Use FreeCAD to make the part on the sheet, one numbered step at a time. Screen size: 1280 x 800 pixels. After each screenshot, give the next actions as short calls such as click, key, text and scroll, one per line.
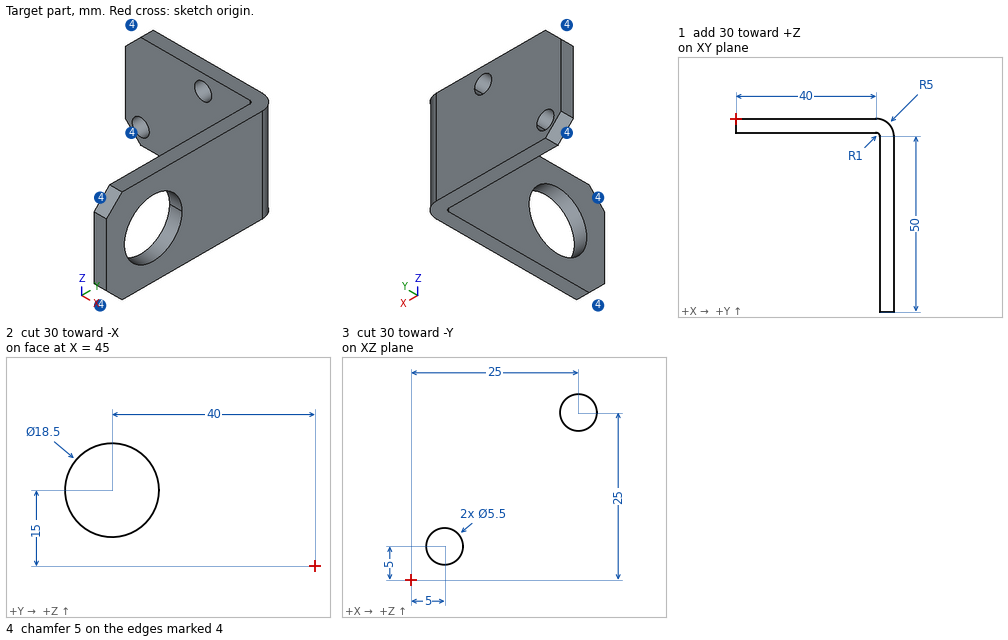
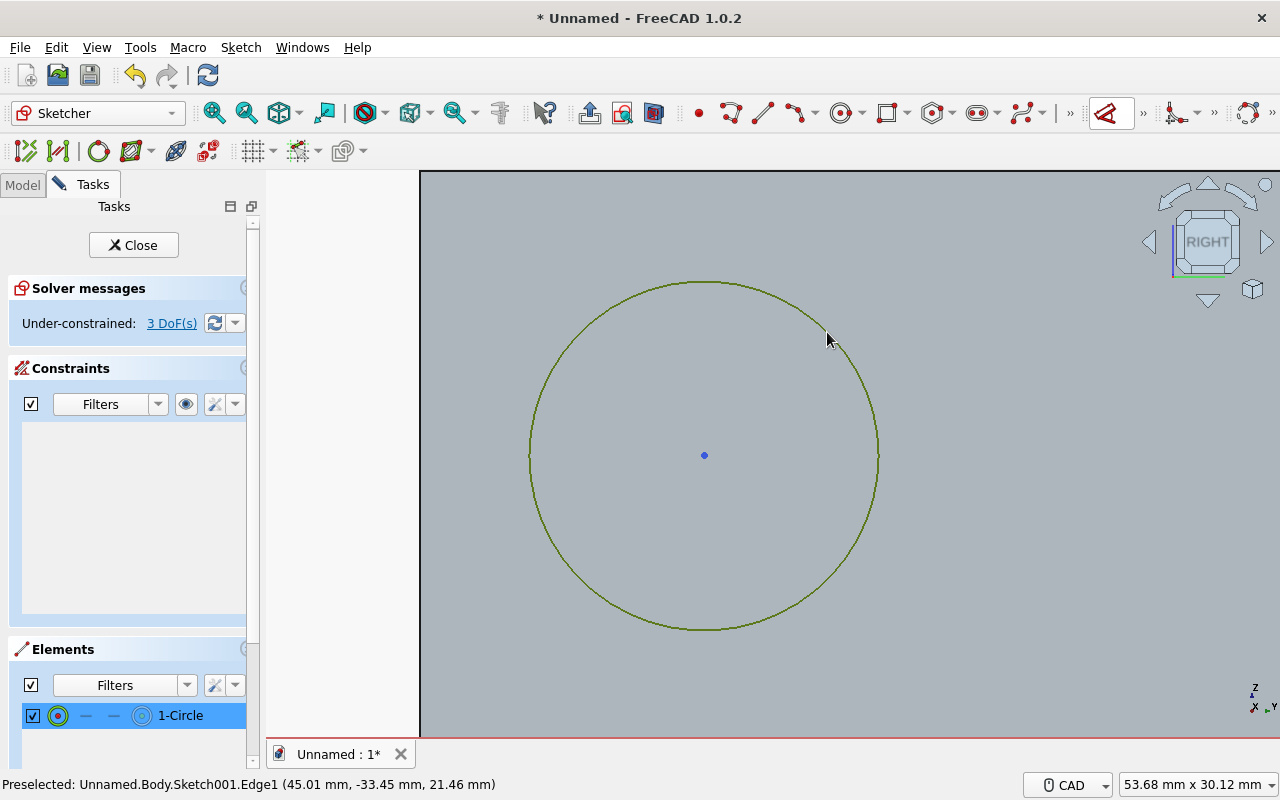
click(1128, 114)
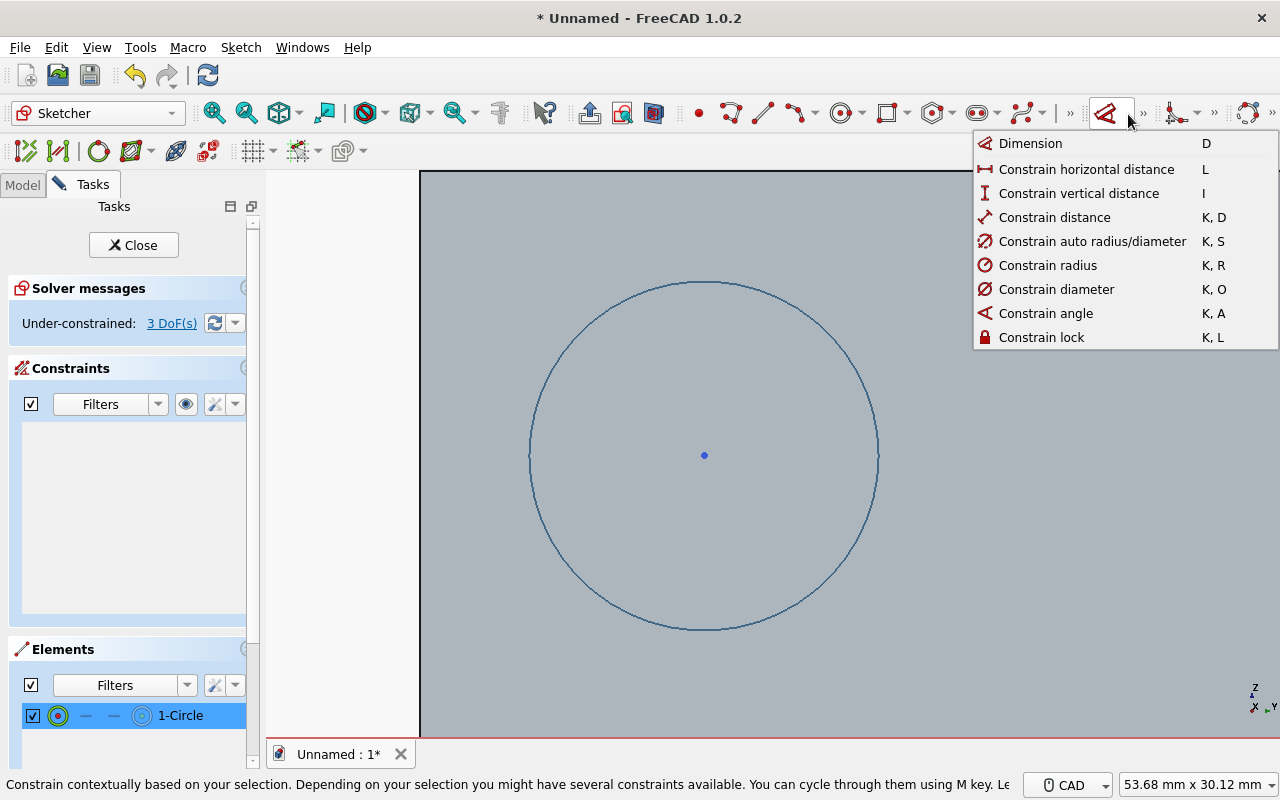
click(1126, 289)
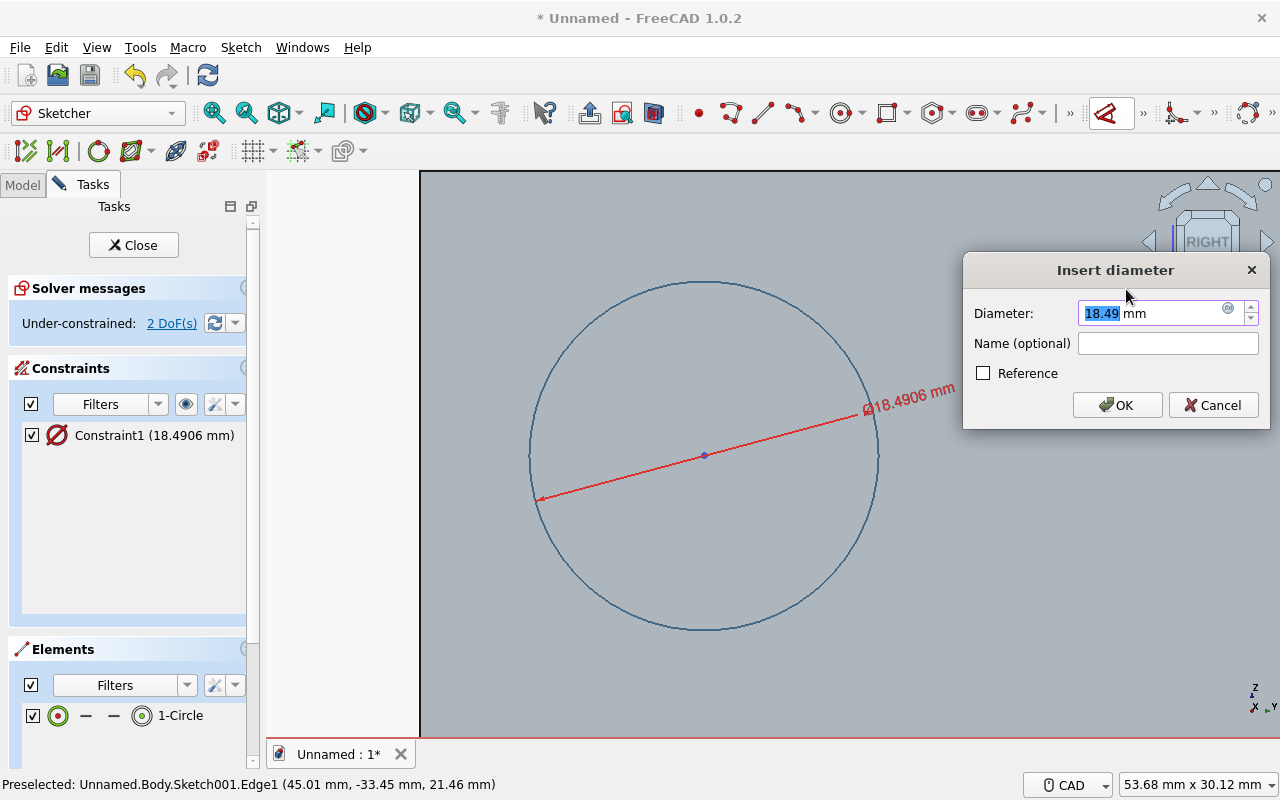
text(18.5)
key(Return)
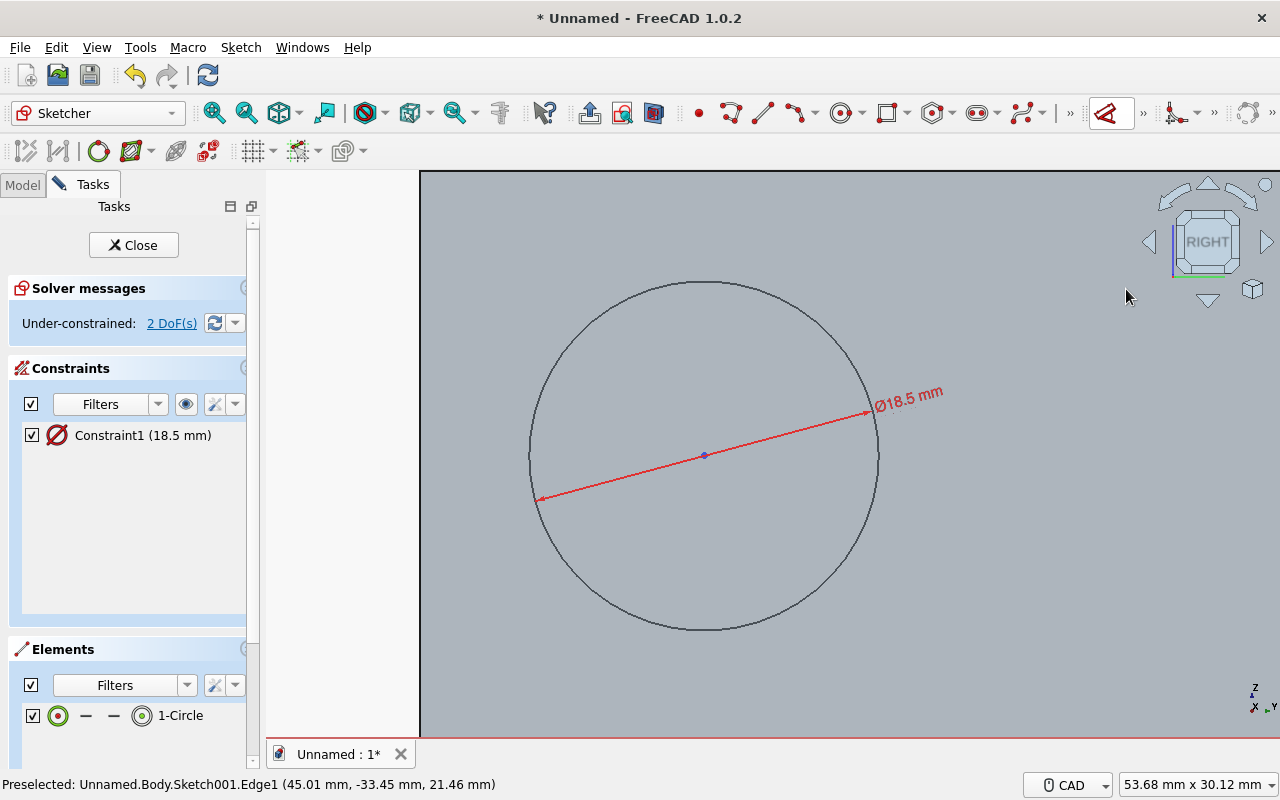
click(704, 456)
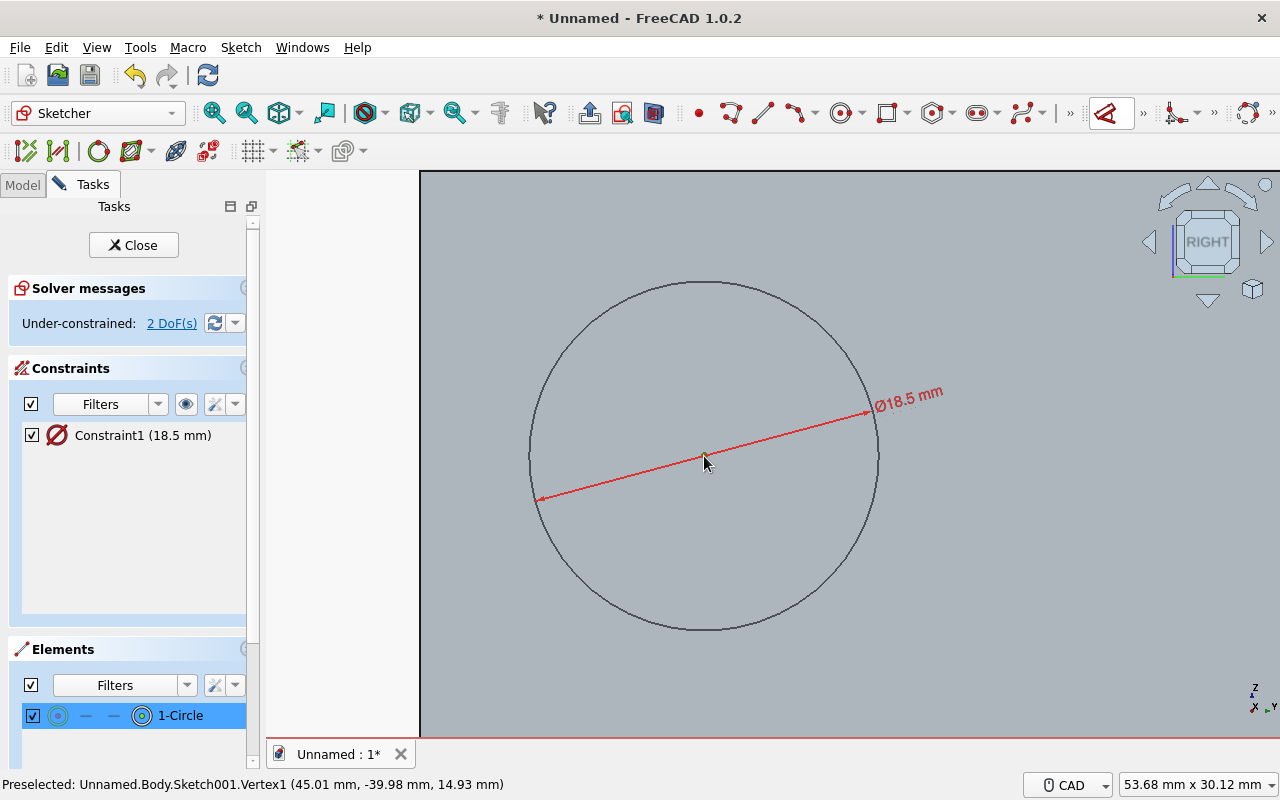
click(1128, 114)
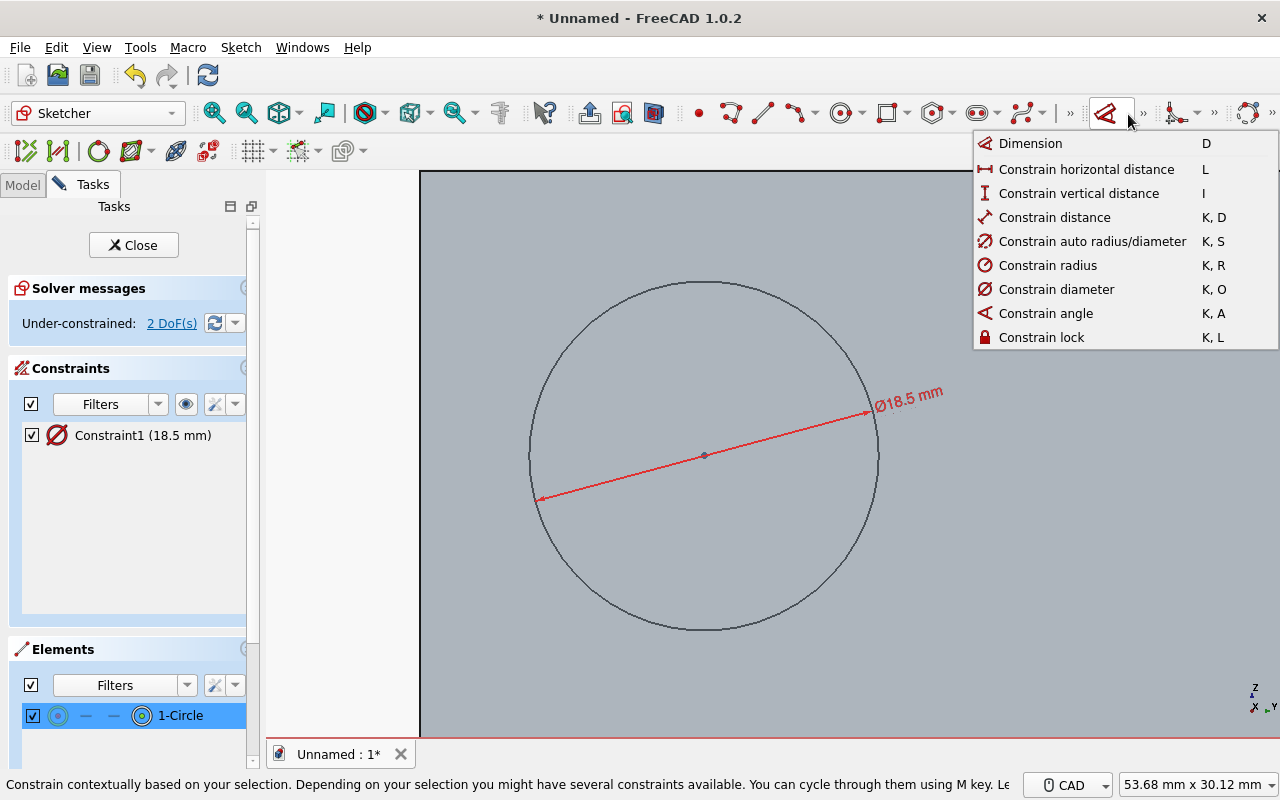
click(1126, 169)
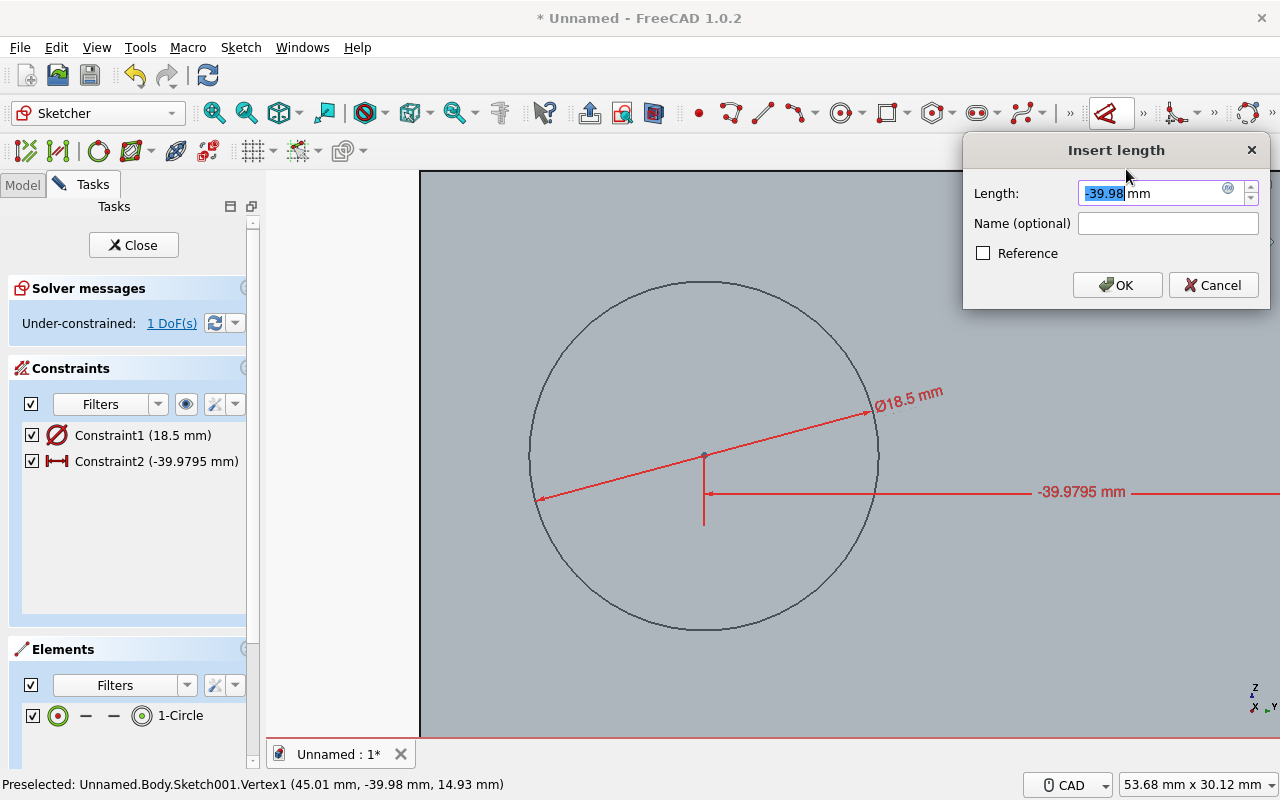
text(-40)
key(Return)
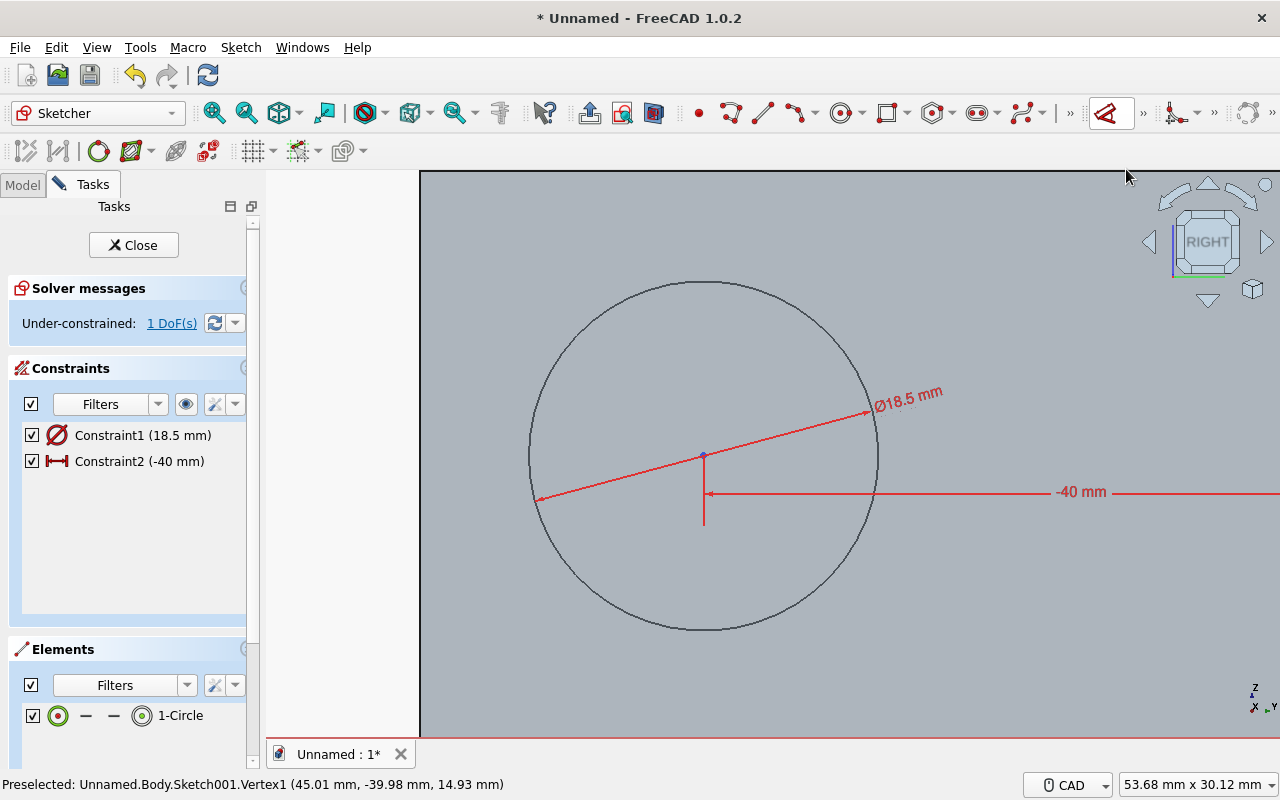
click(704, 456)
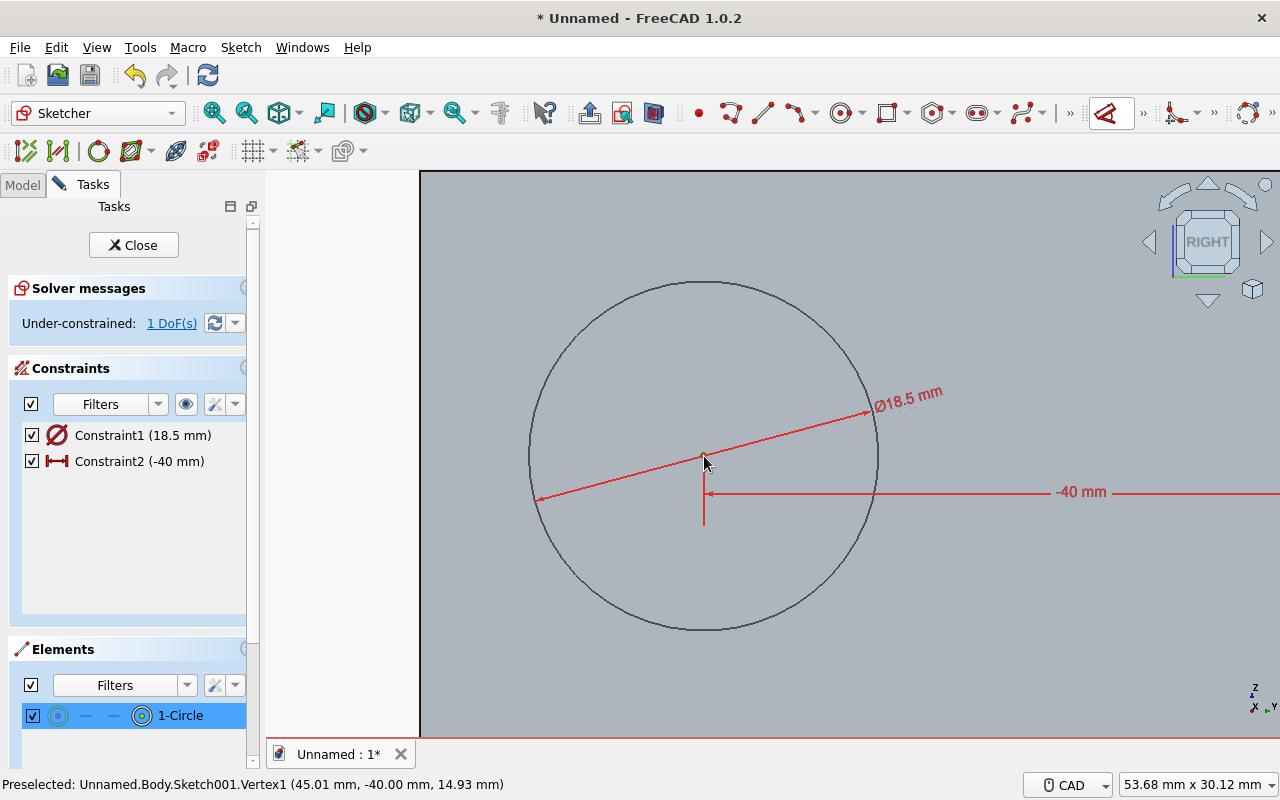
key(i)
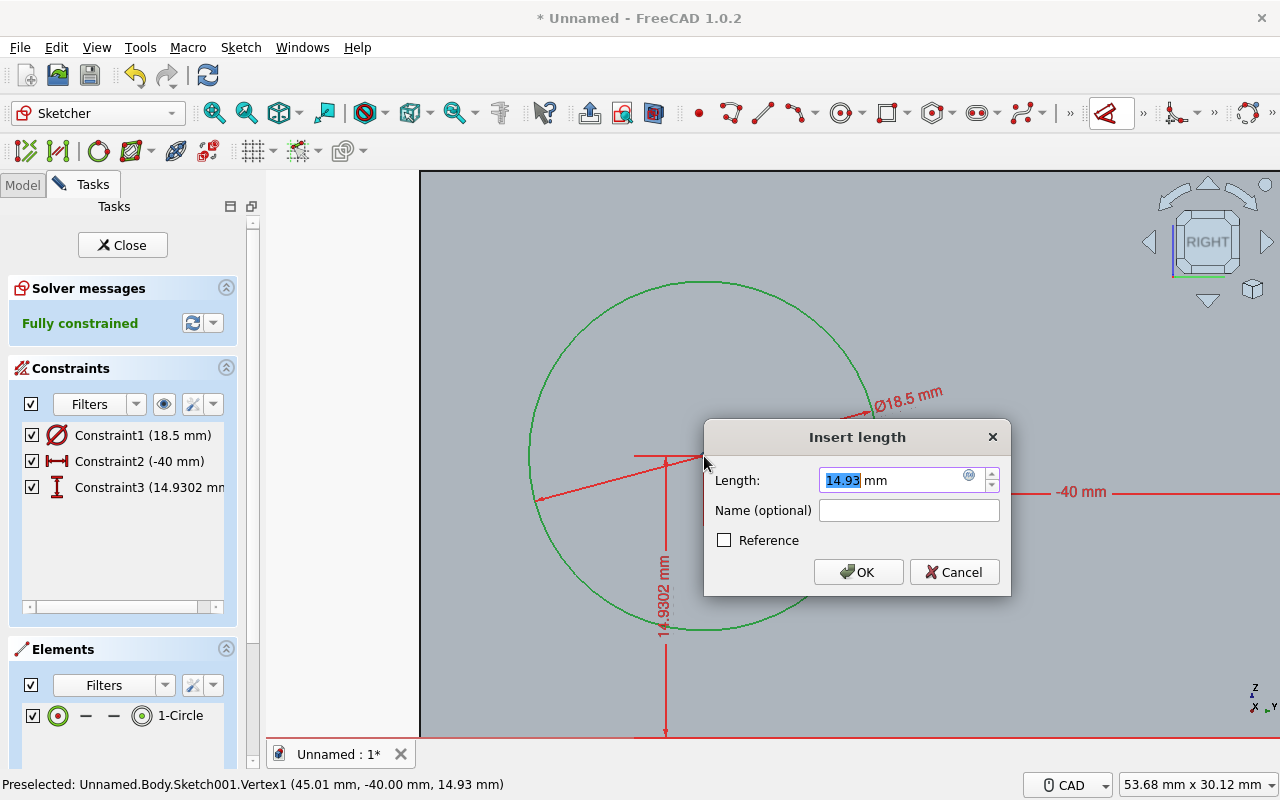
text(15)
key(Return)